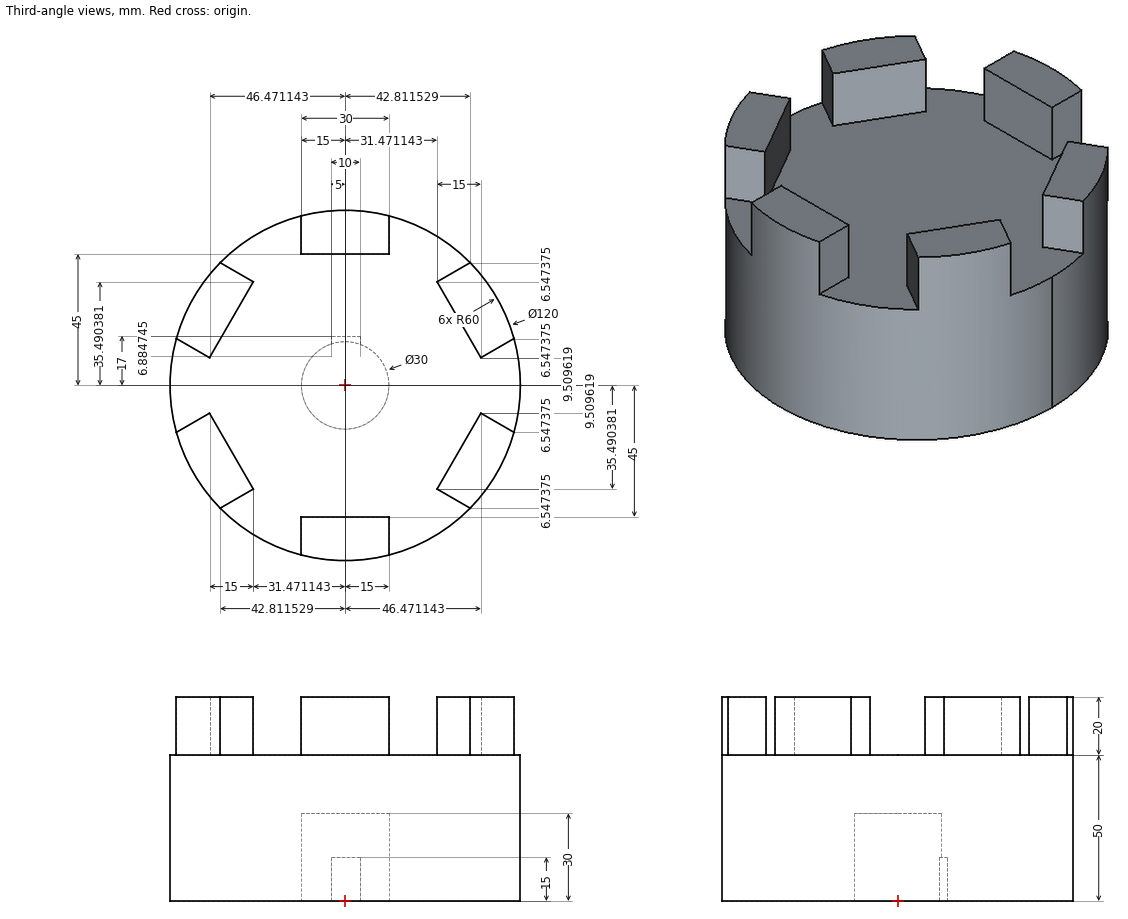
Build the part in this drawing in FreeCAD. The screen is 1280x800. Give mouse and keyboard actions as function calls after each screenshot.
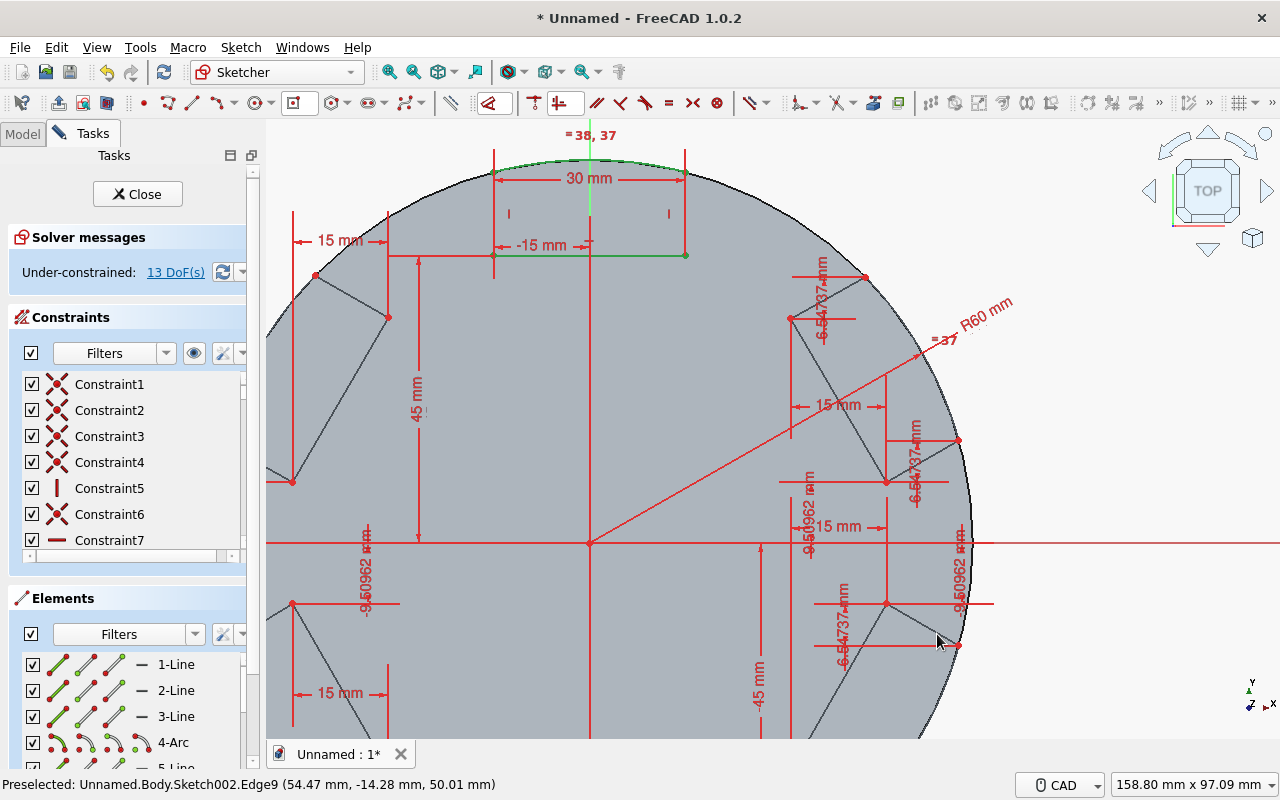
scroll(844, 290, down, 3)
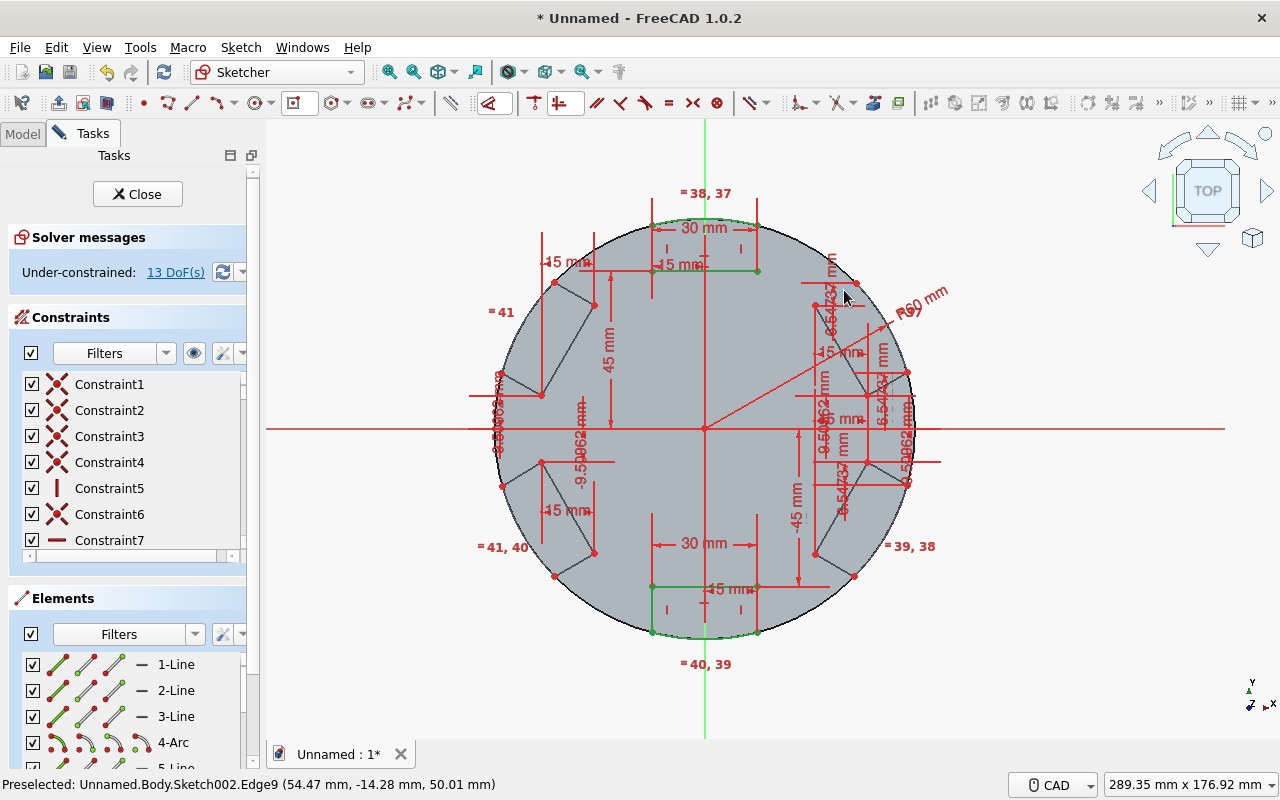
scroll(827, 561, up, 3)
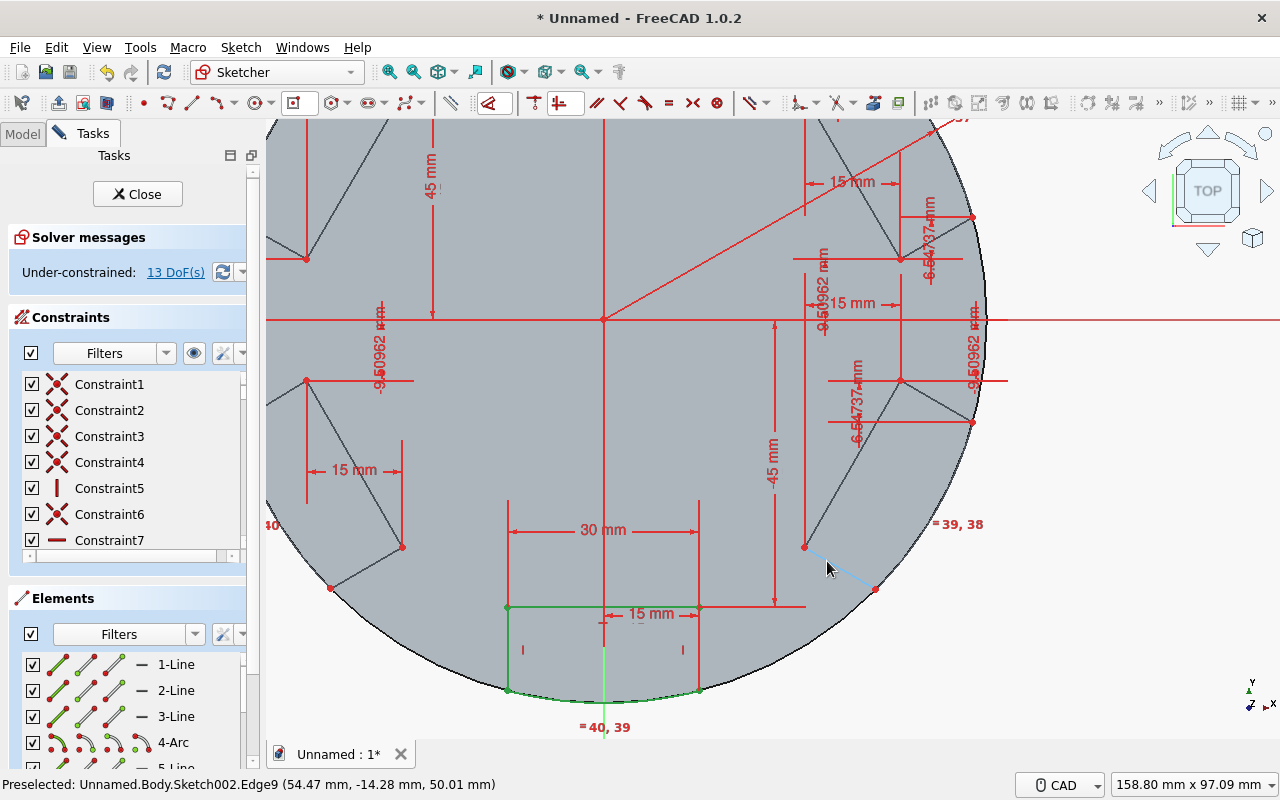
click(826, 560)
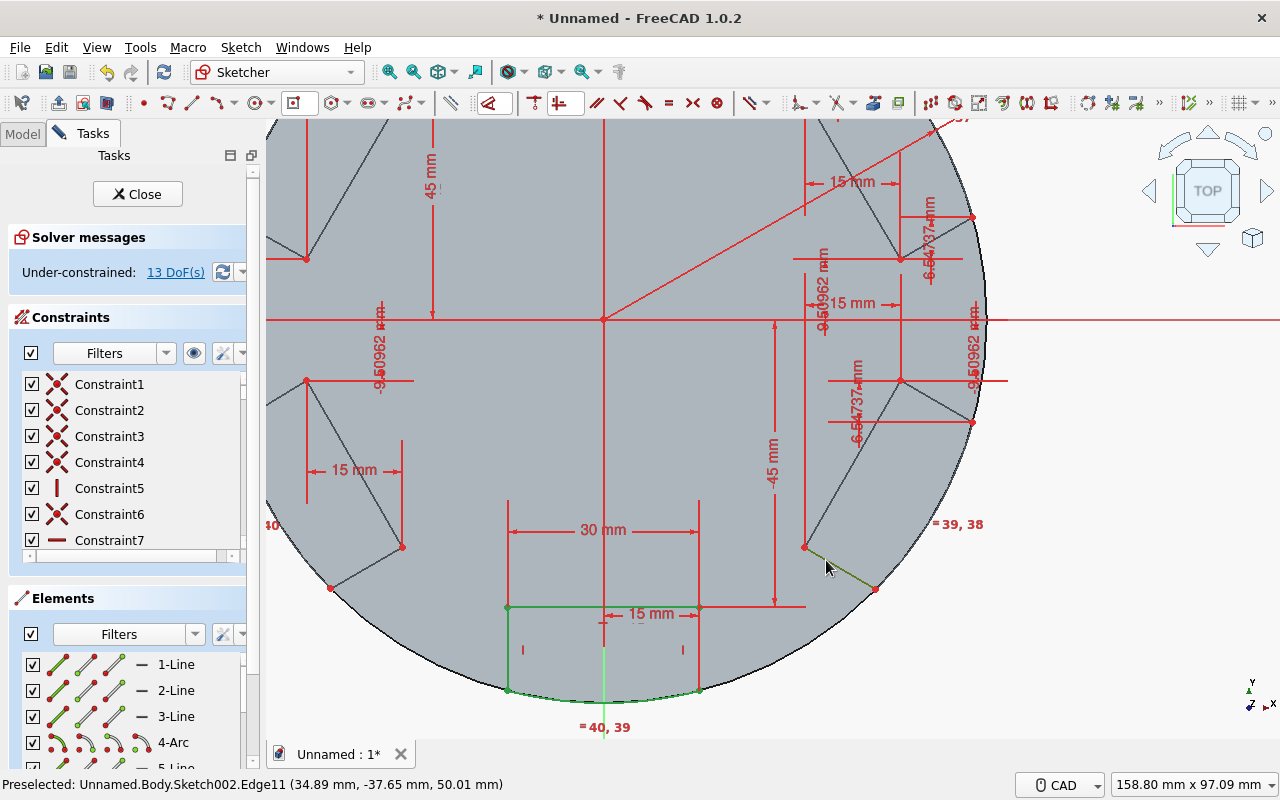
key(i)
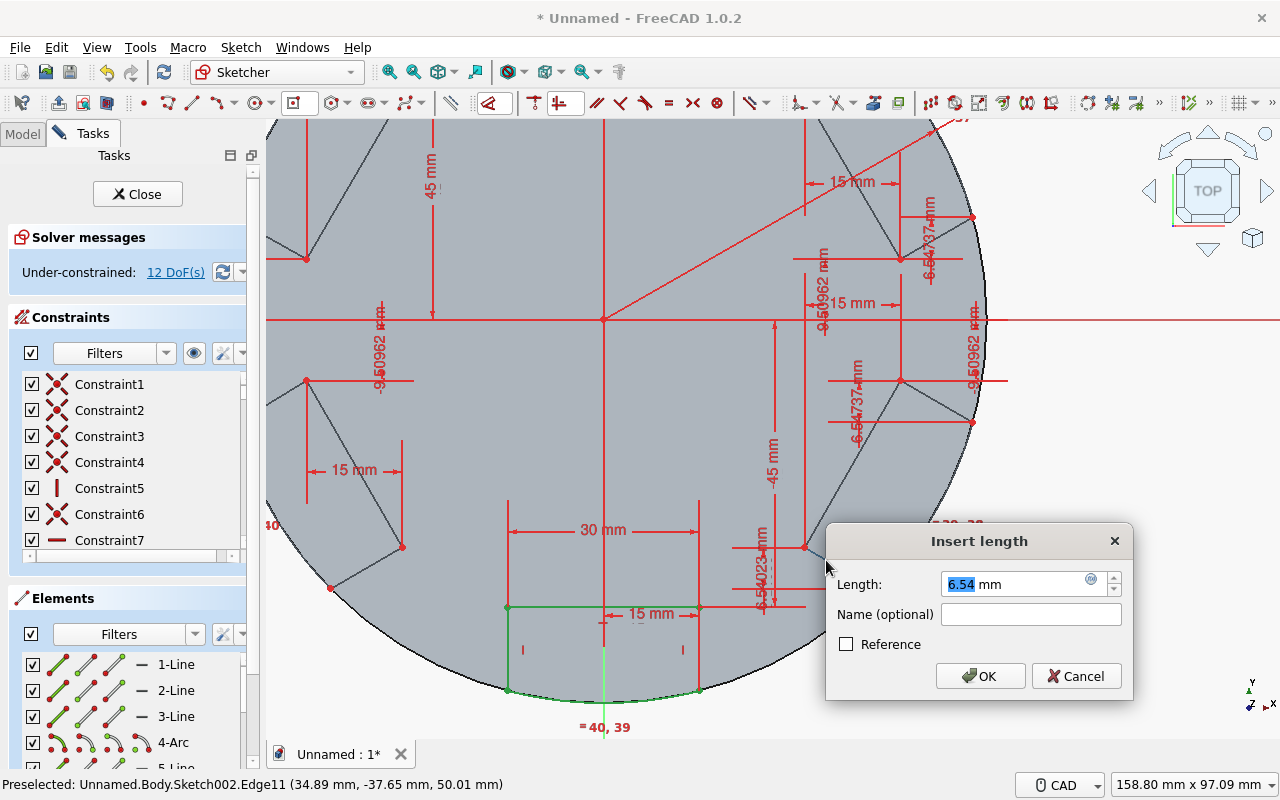
text(6.547375)
key(Return)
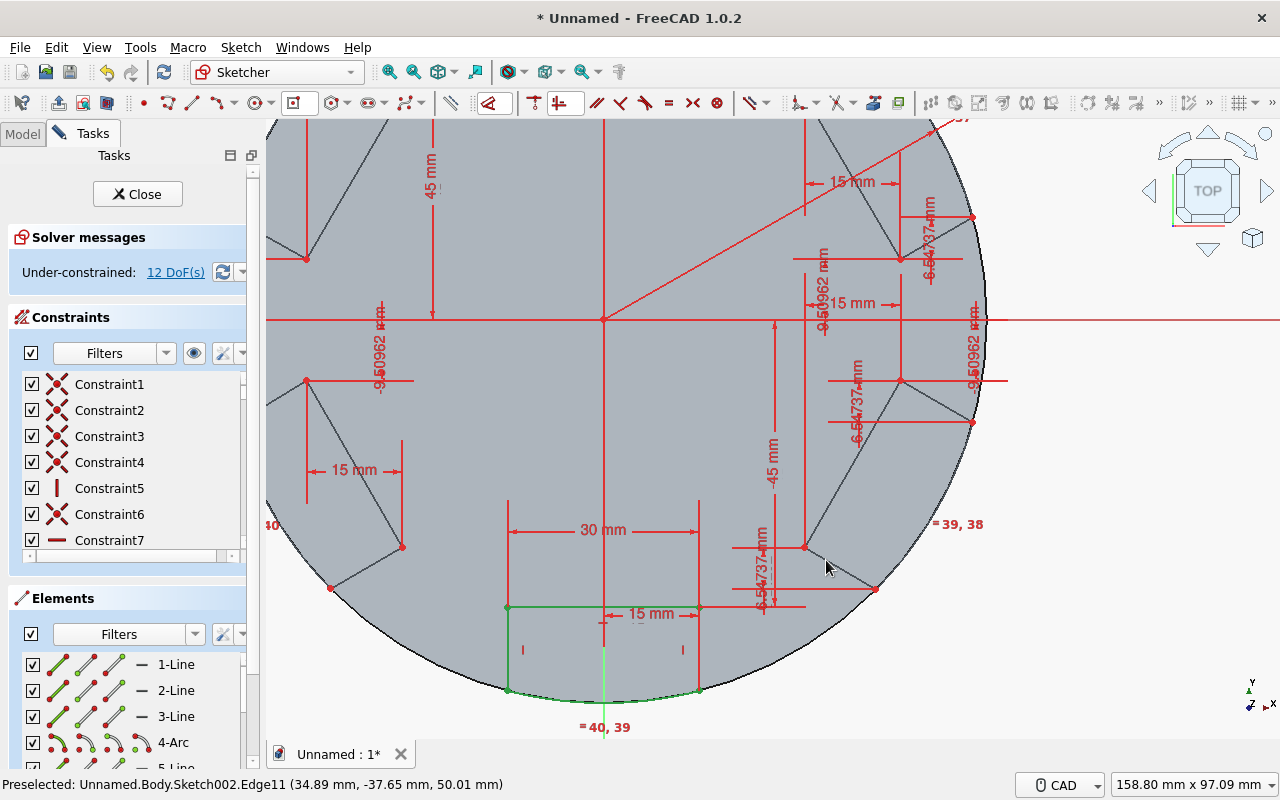
click(352, 576)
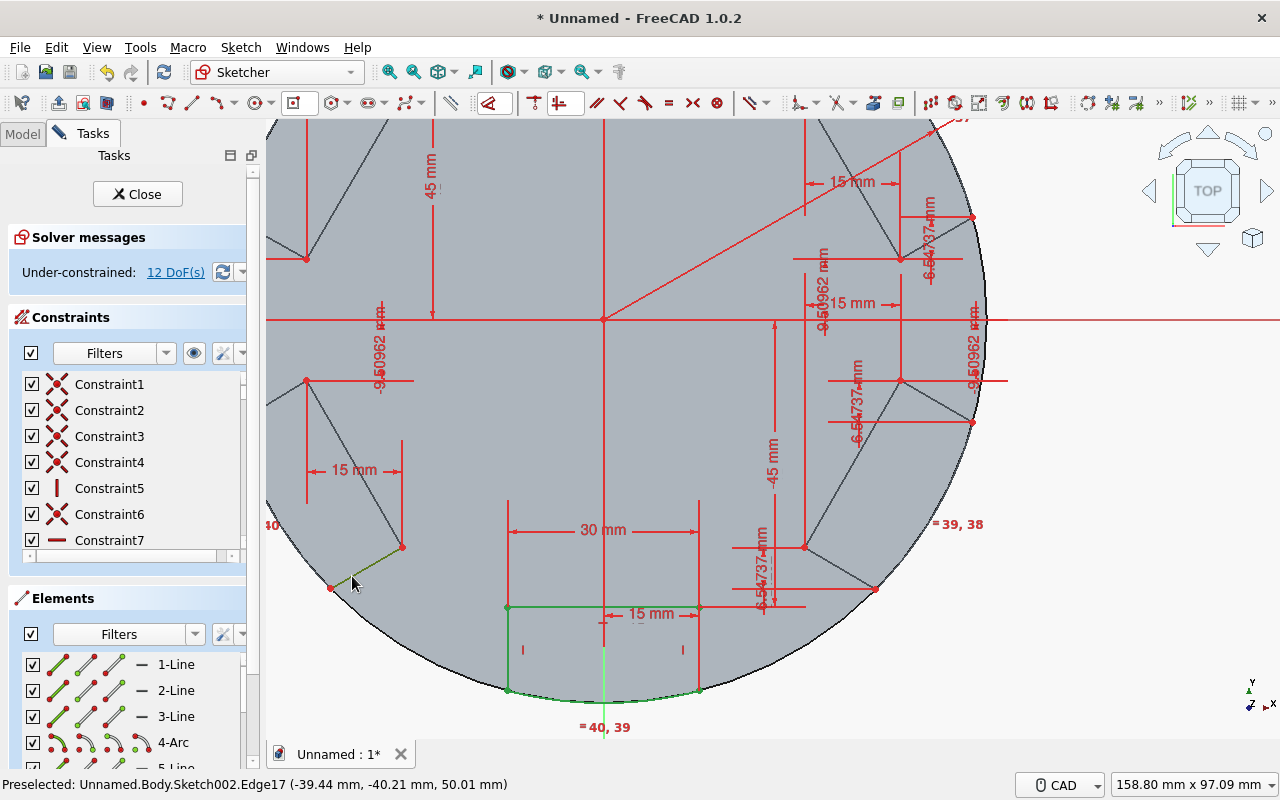
key(i)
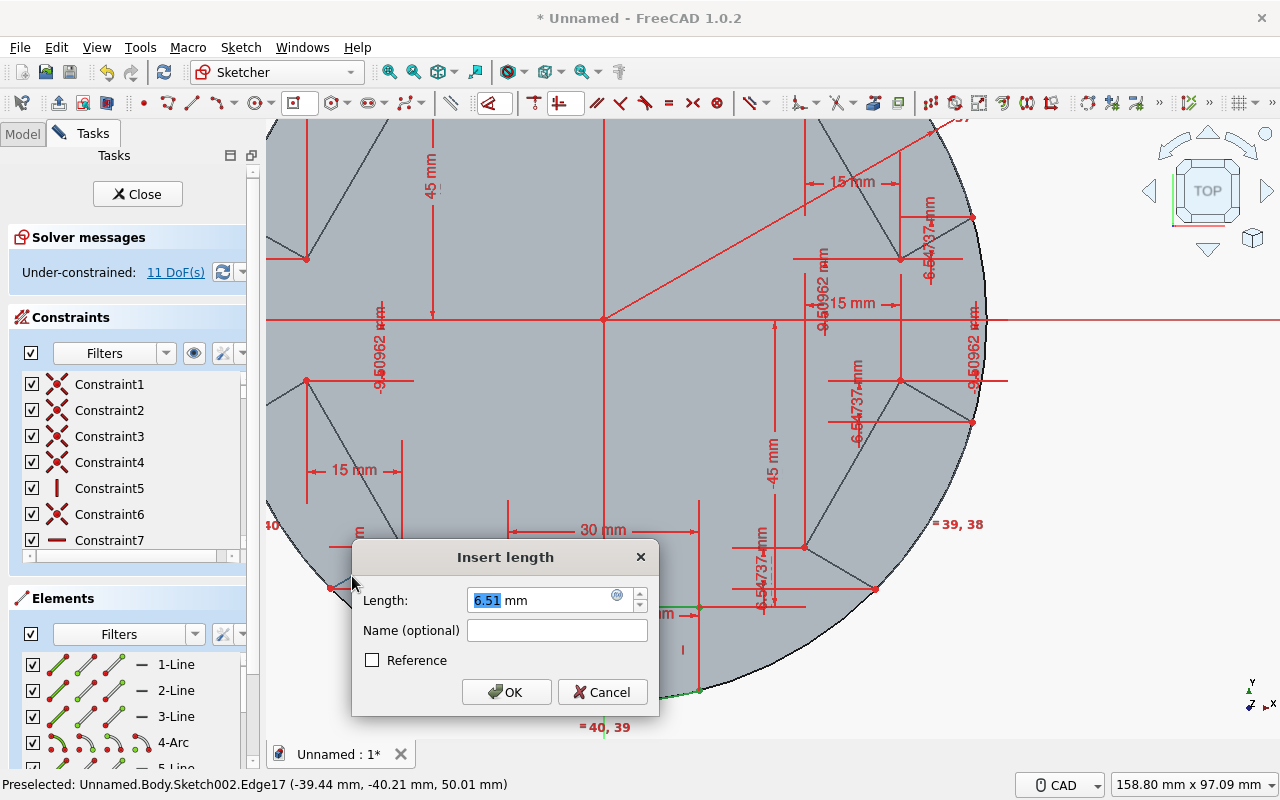
text(6.547375)
key(Return)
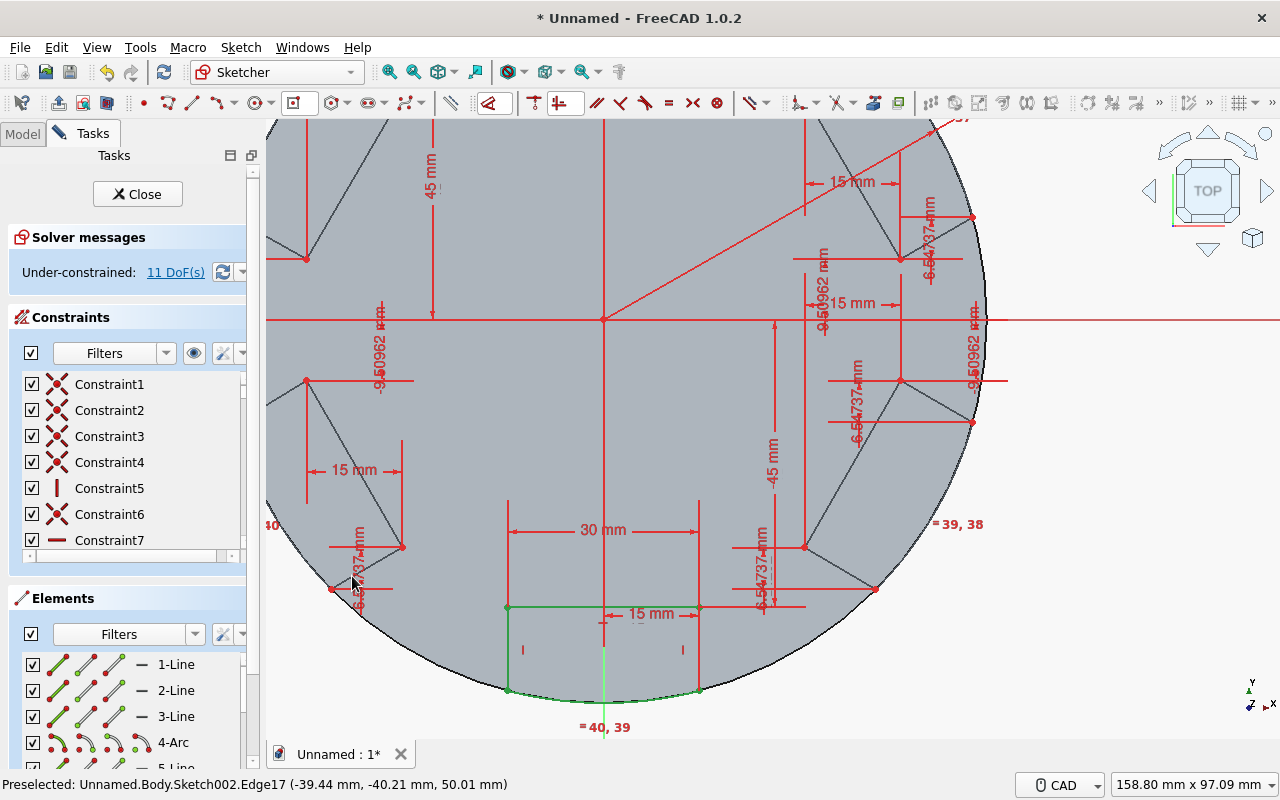
scroll(827, 562, down, 3)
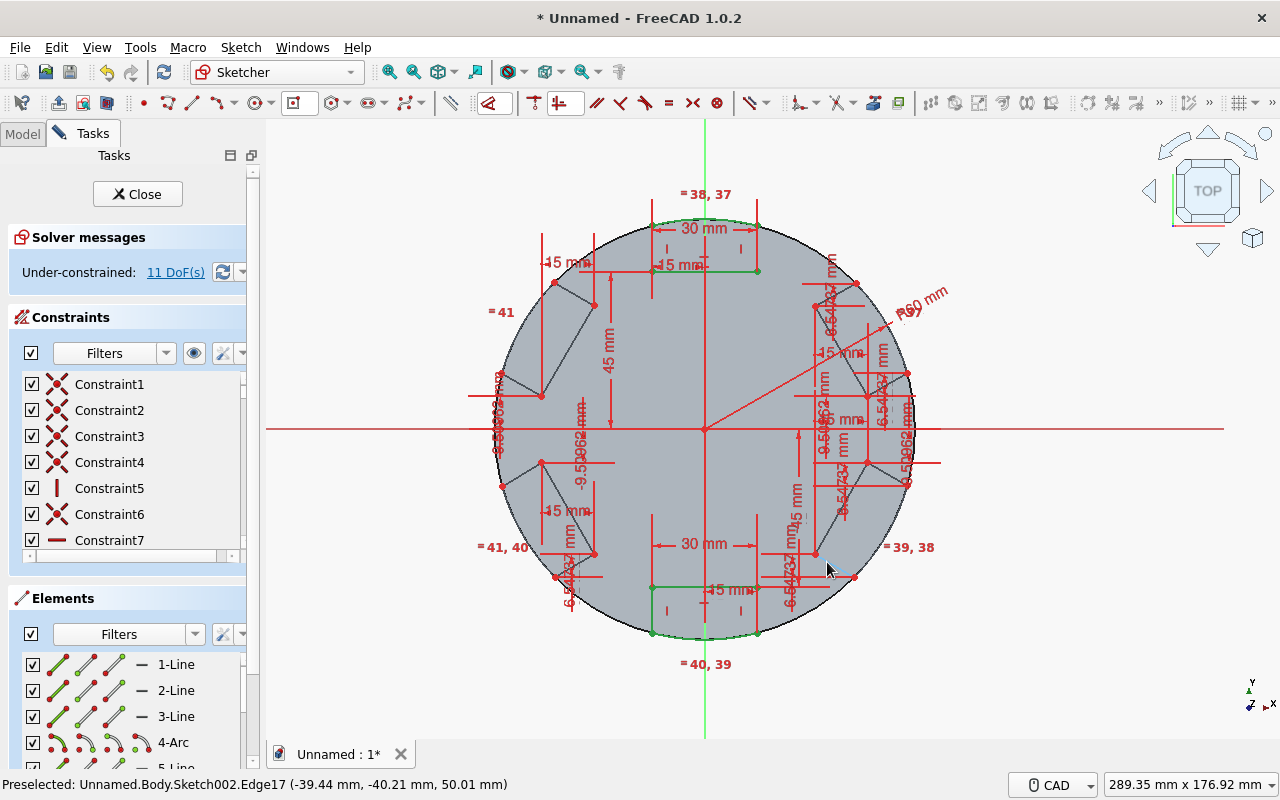
scroll(530, 470, up, 3)